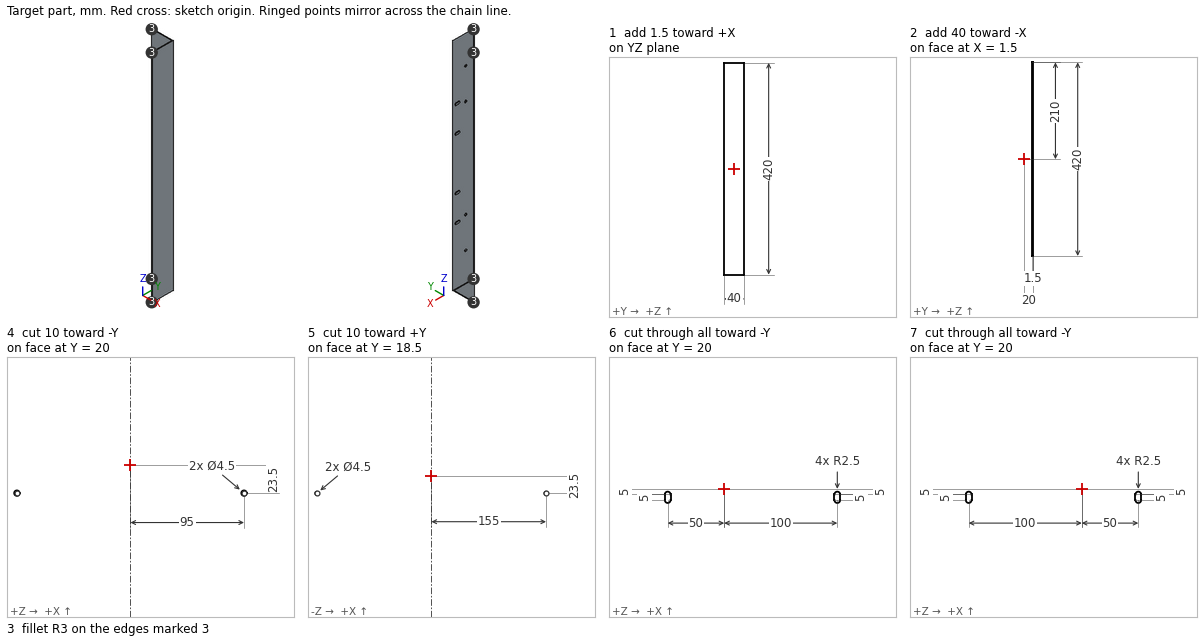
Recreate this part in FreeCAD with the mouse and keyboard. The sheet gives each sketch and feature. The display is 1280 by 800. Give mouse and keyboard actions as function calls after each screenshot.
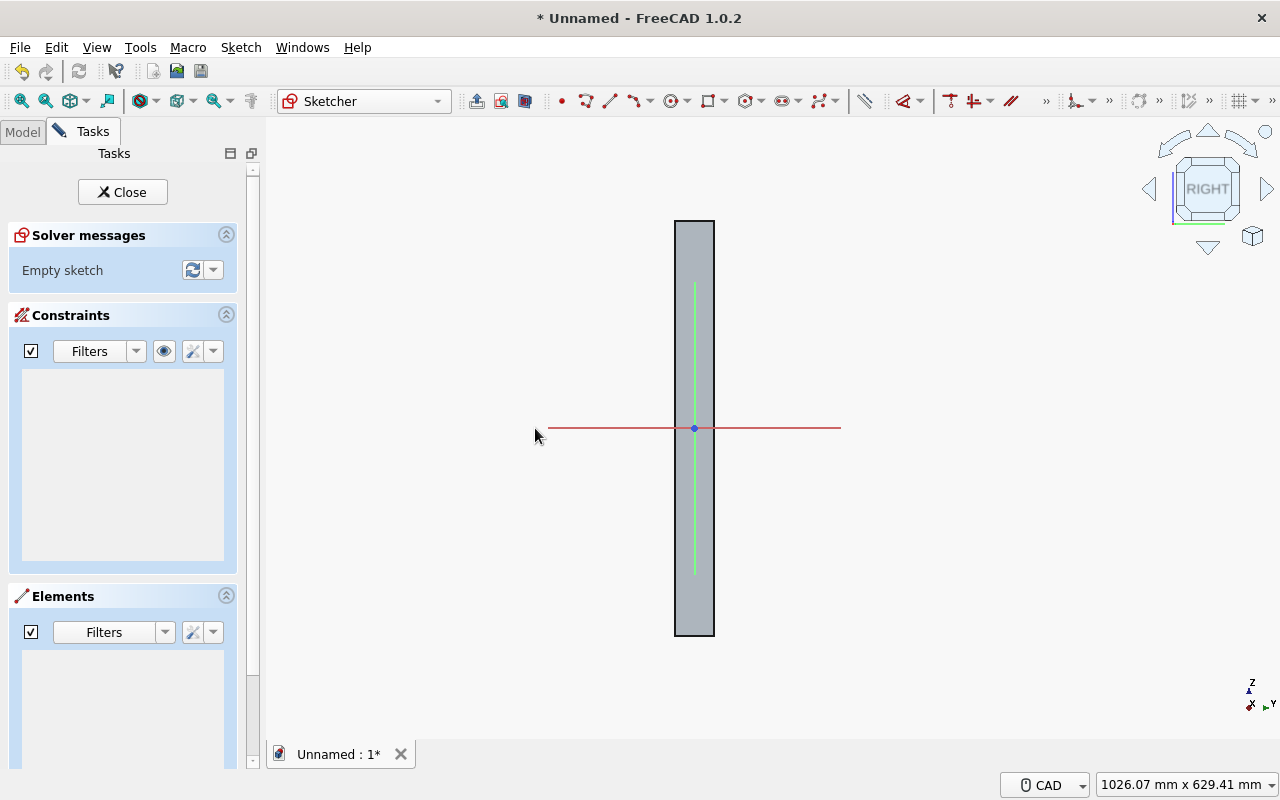
click(708, 102)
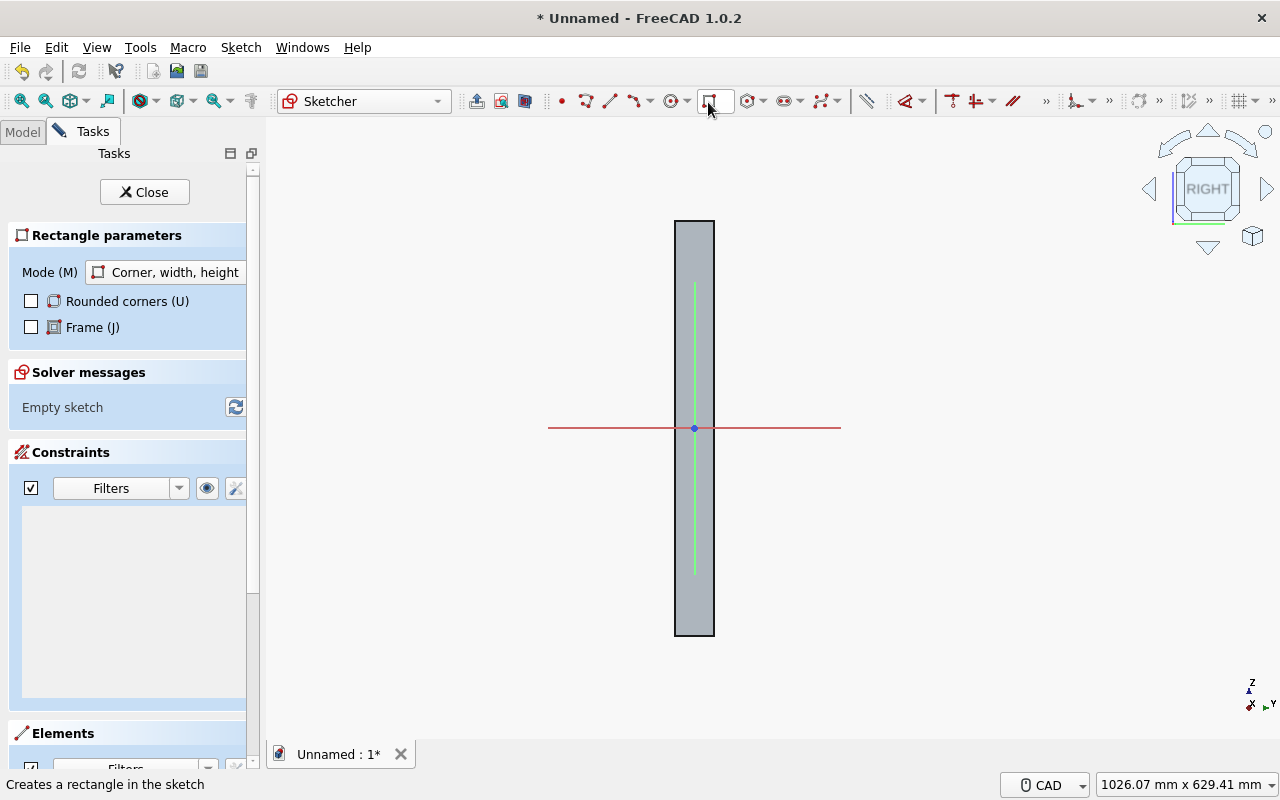
scroll(713, 221, up, 12)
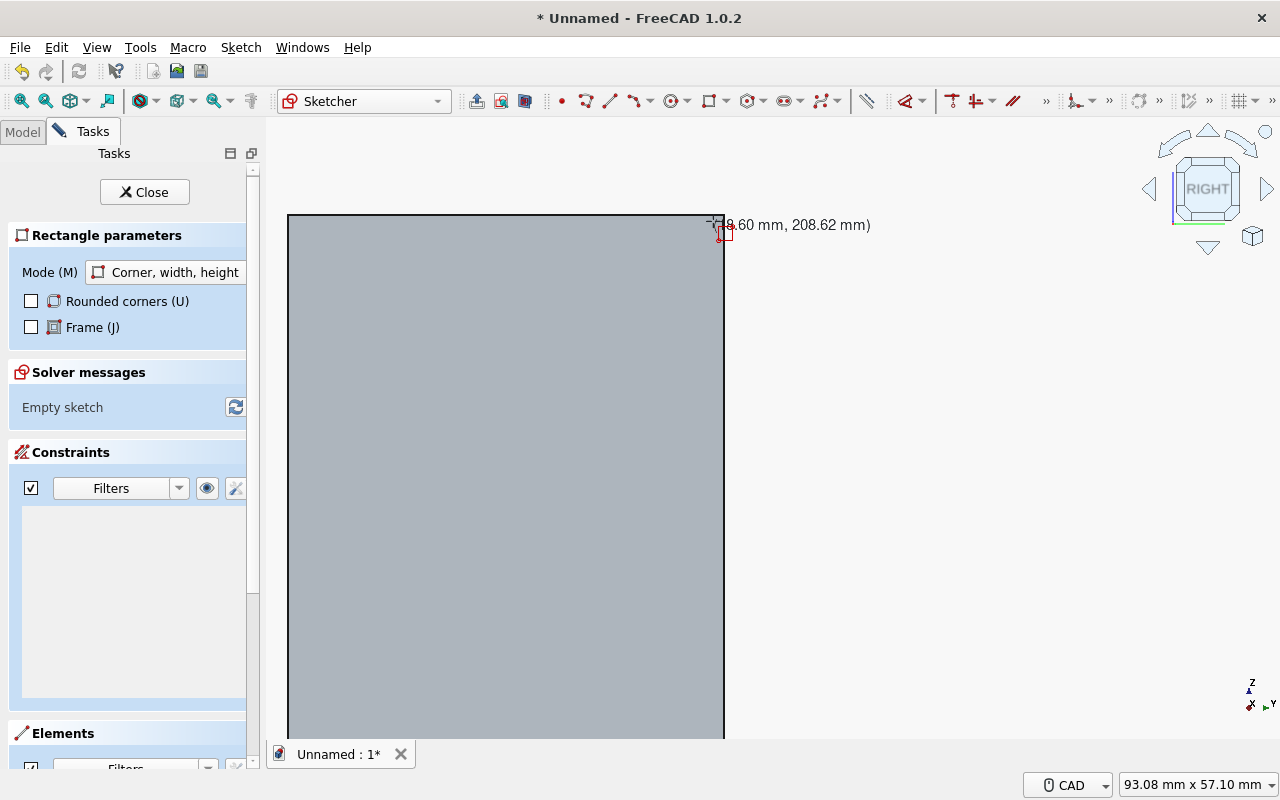
scroll(713, 221, down, 12)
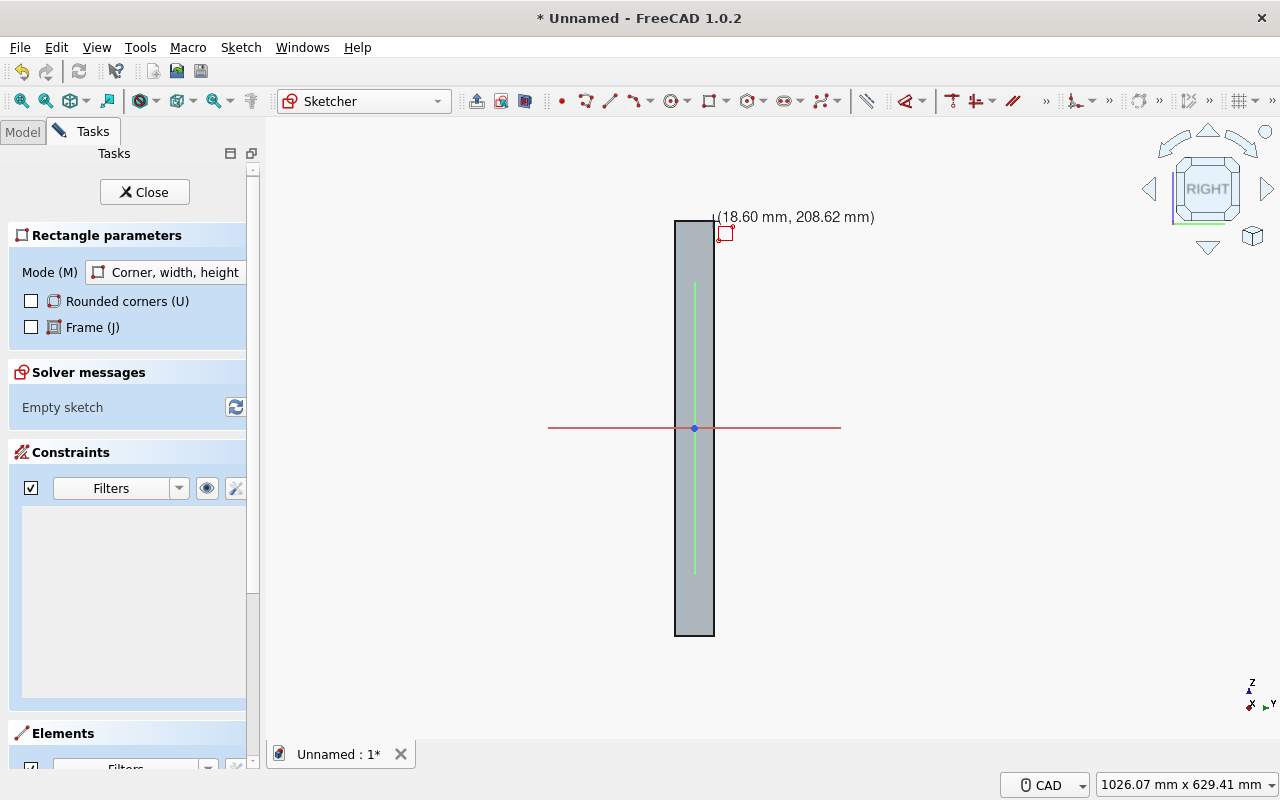
click(713, 221)
click(714, 636)
key(Escape)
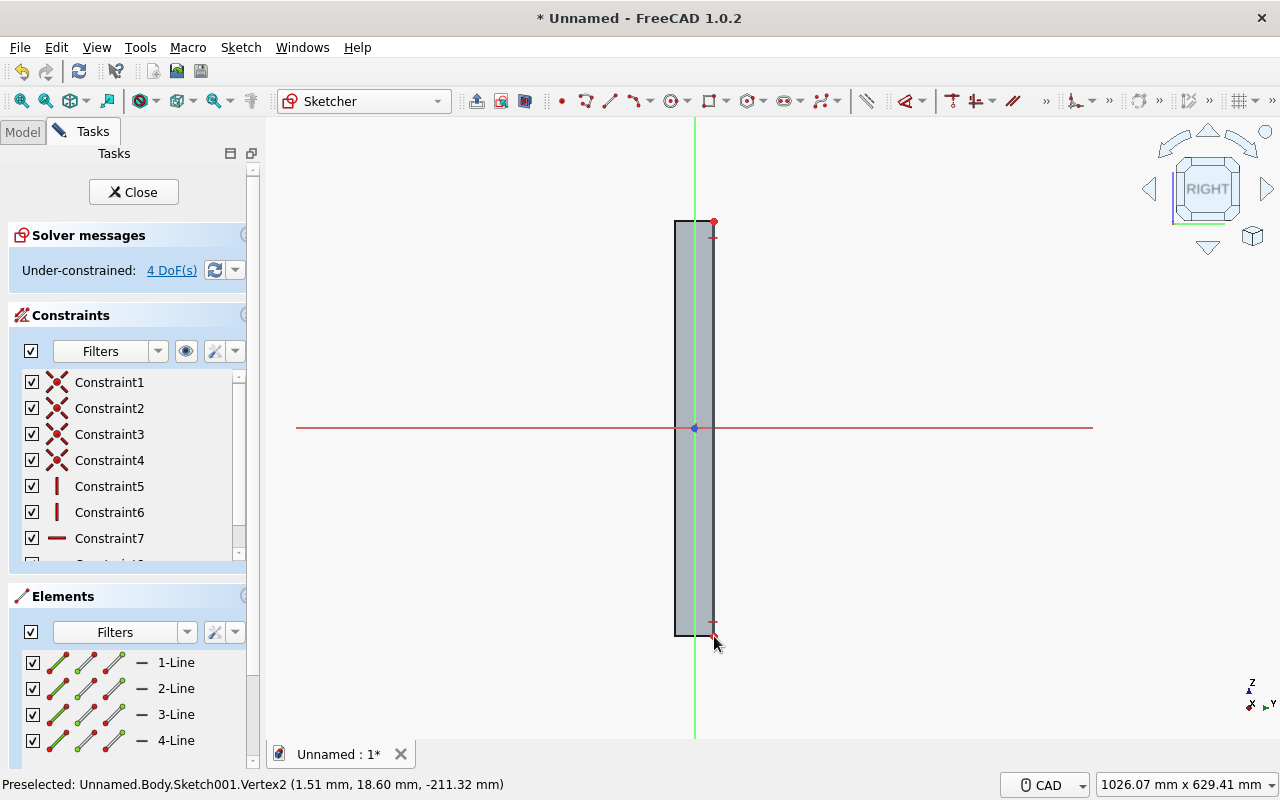
click(906, 102)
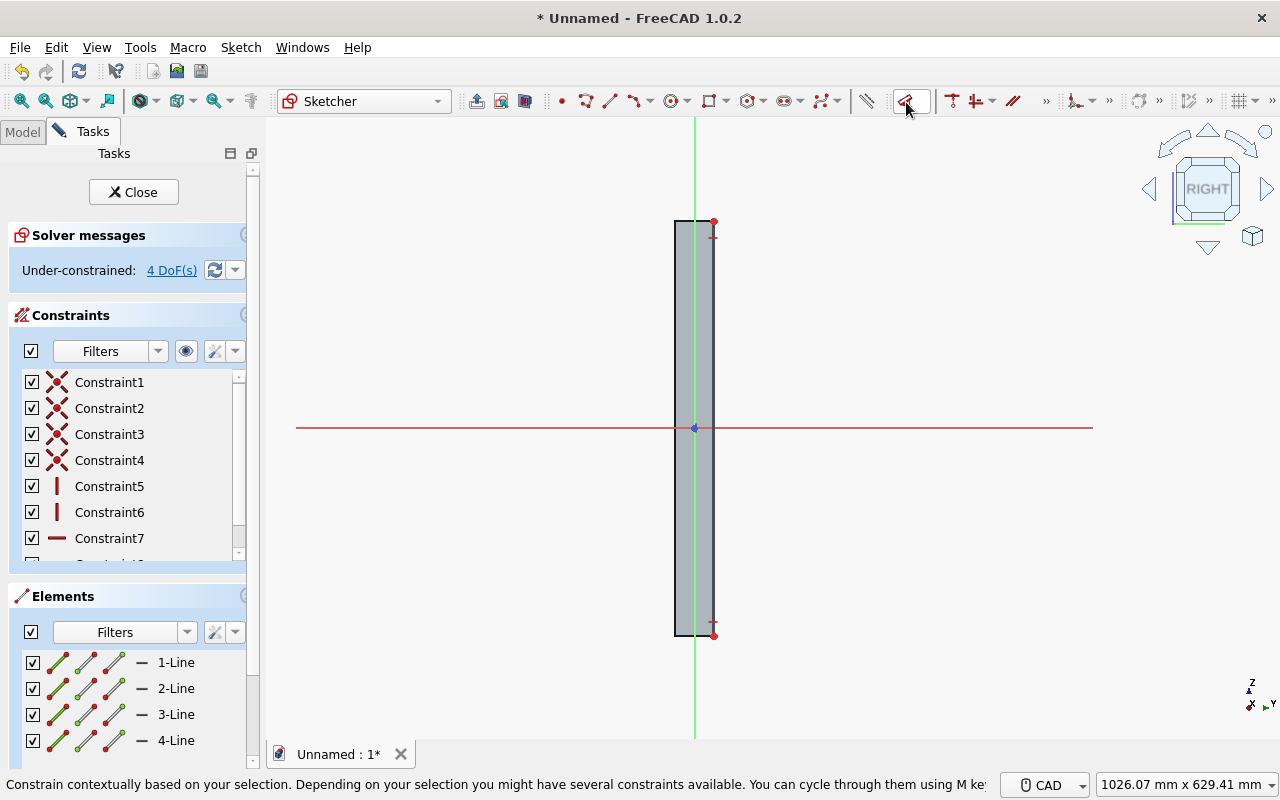
scroll(713, 347, up, 14)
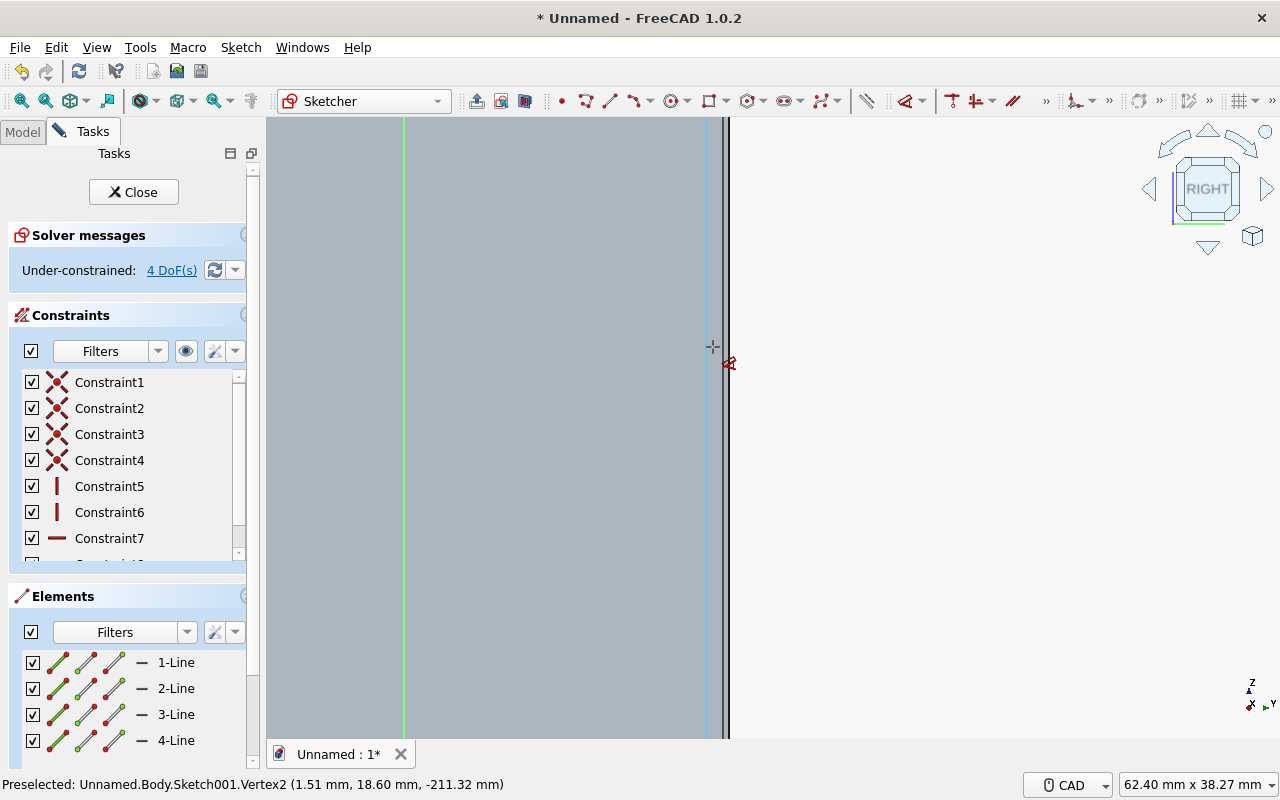
click(706, 333)
click(740, 428)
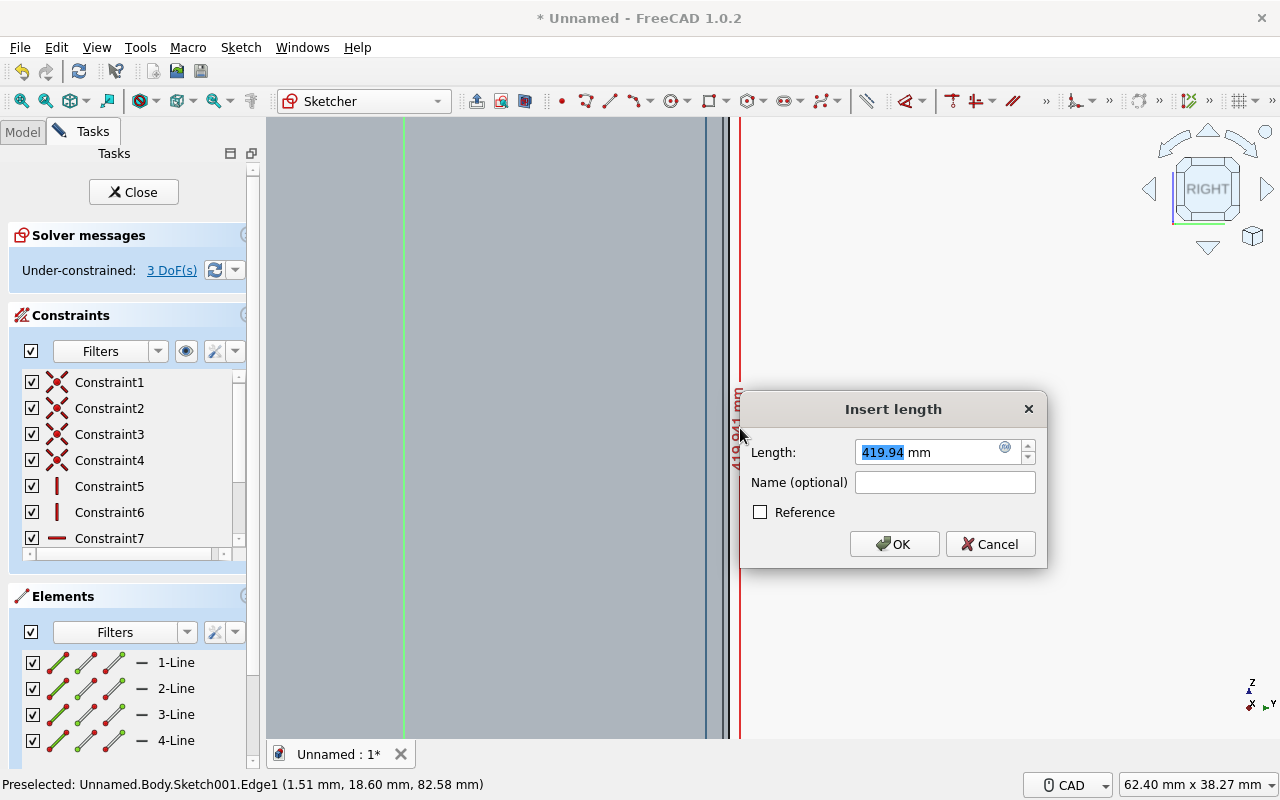
text(420)
key(Return)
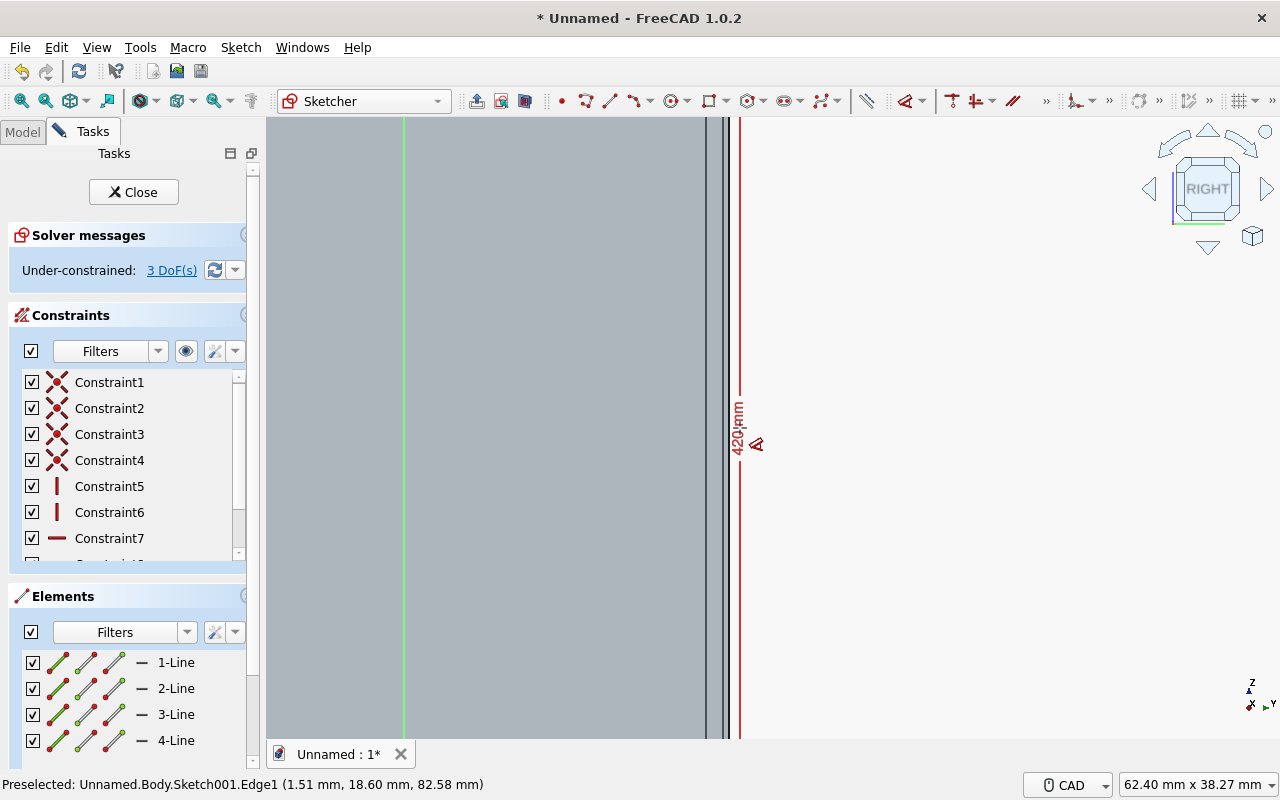
scroll(713, 347, down, 14)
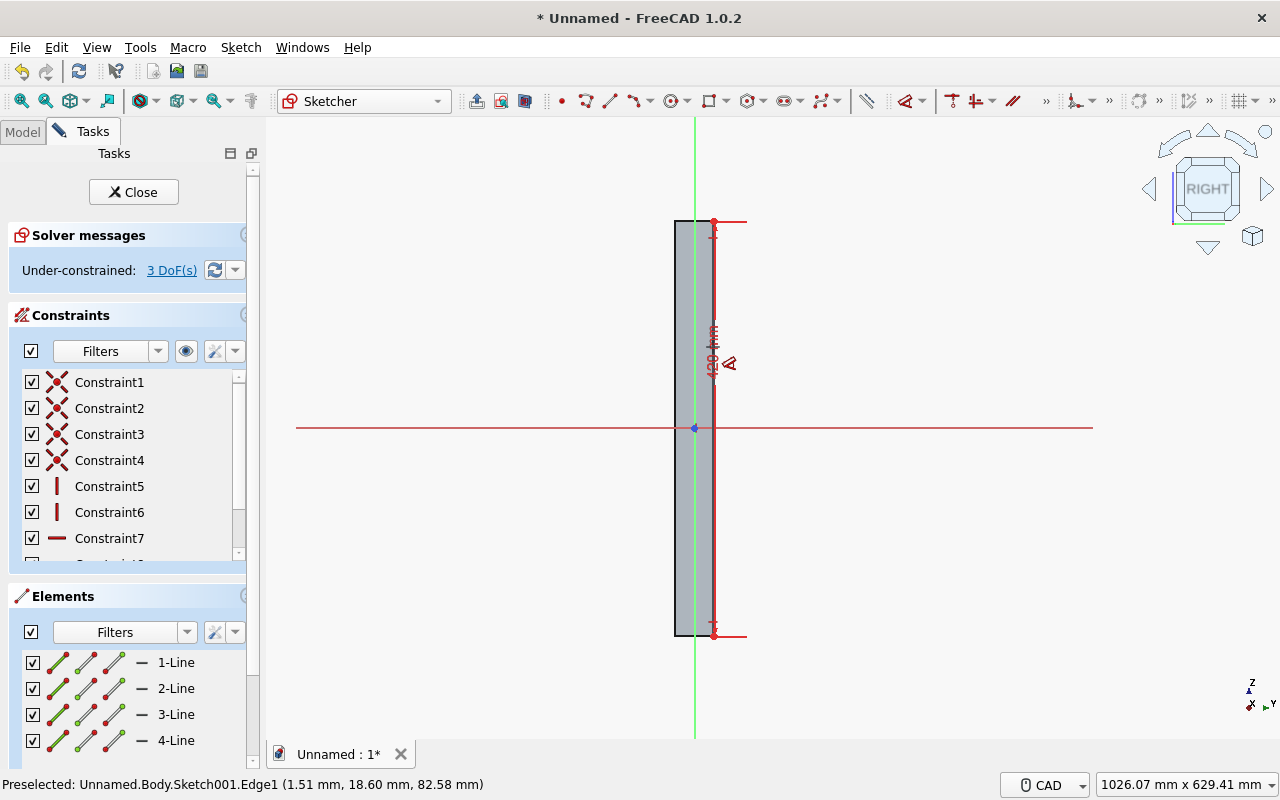
scroll(714, 637, up, 17)